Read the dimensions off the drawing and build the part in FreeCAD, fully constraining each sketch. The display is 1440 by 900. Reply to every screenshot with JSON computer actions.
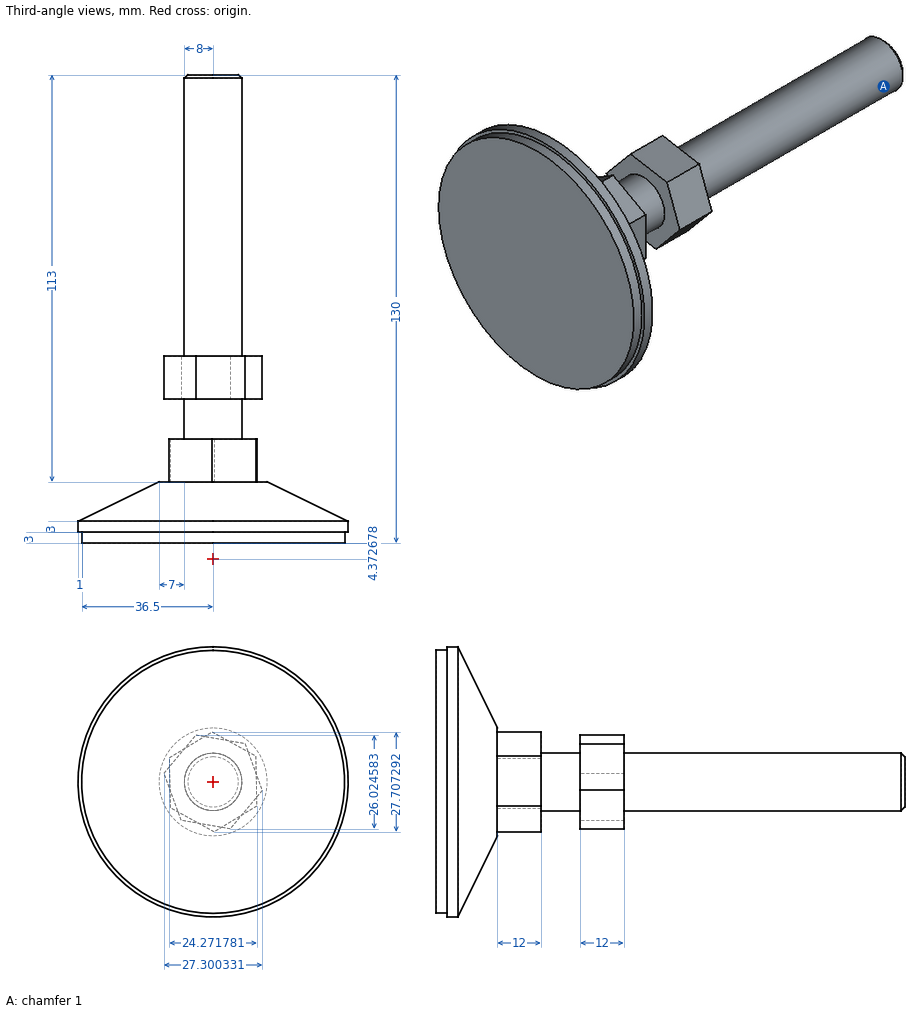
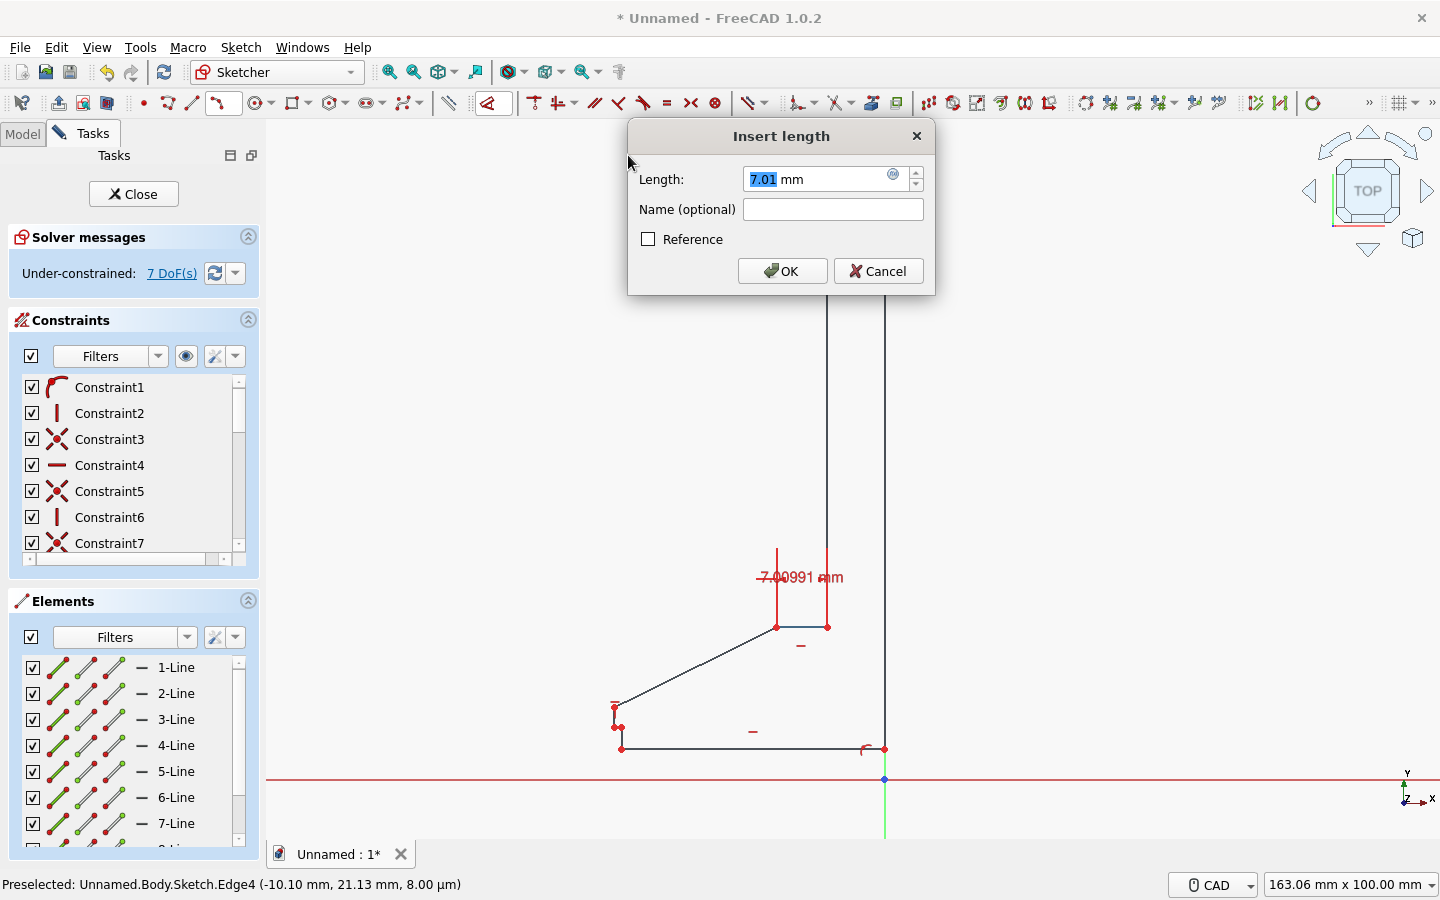
{"action": "type", "text": "7"}
{"action": "key", "text": "Return"}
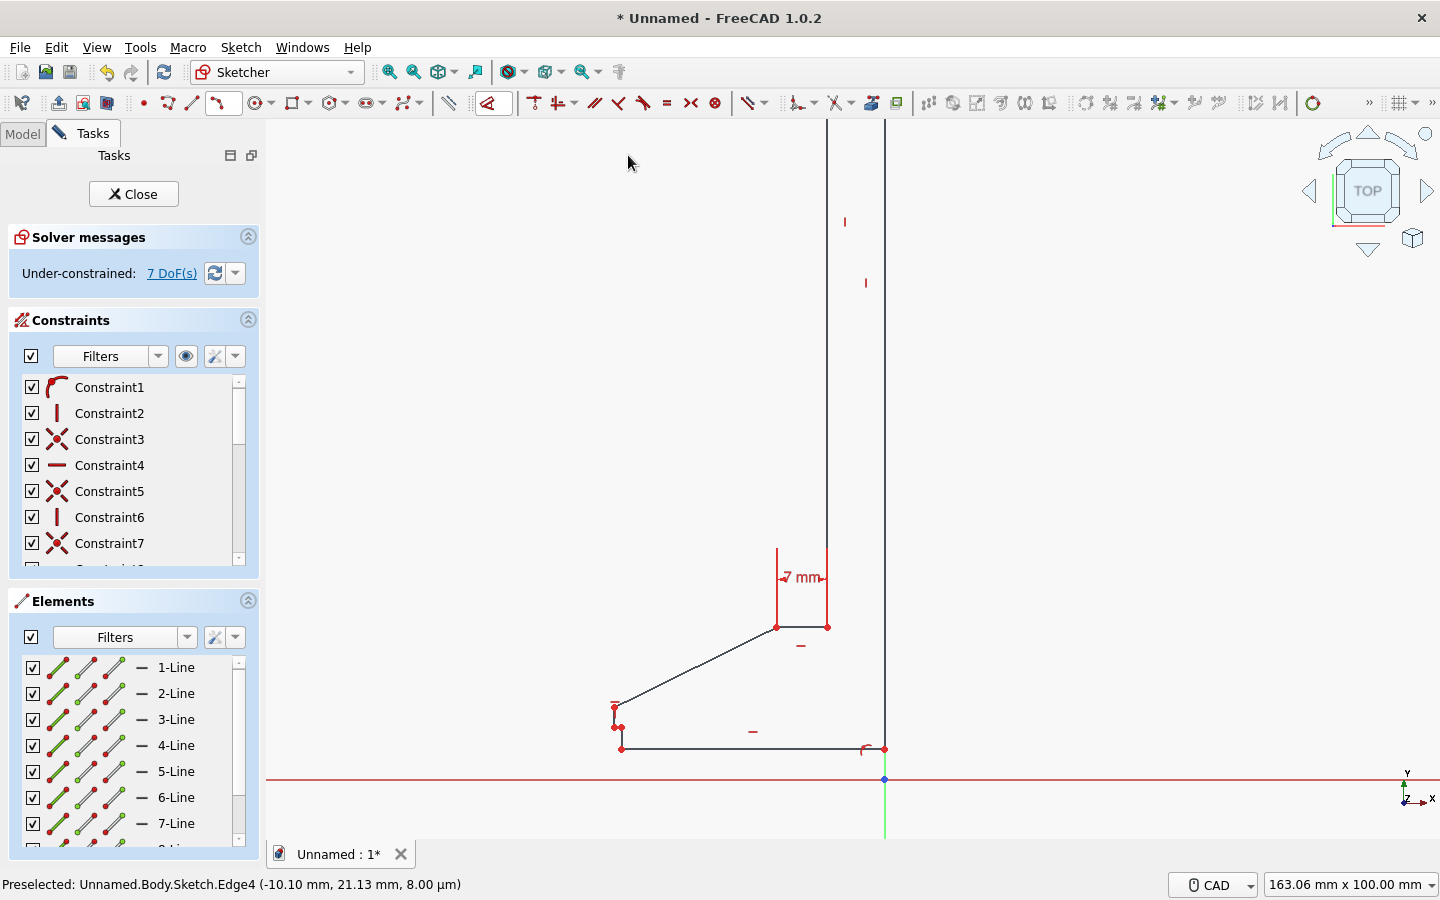
{"action": "scroll", "coordinate": [614, 717], "scroll_direction": "up", "scroll_amount": 4}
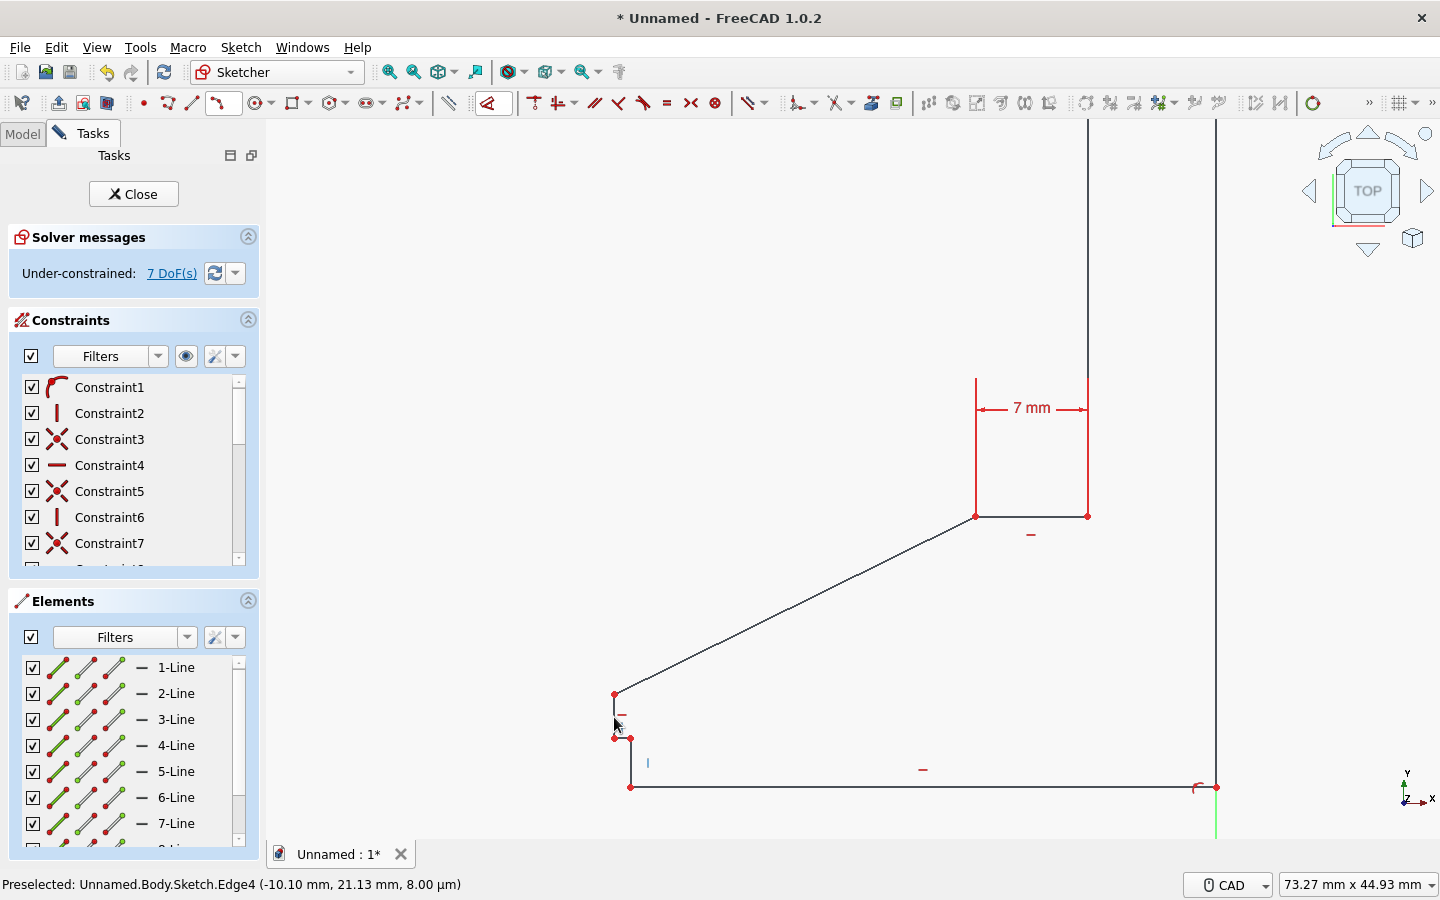
{"action": "left_click", "coordinate": [614, 717]}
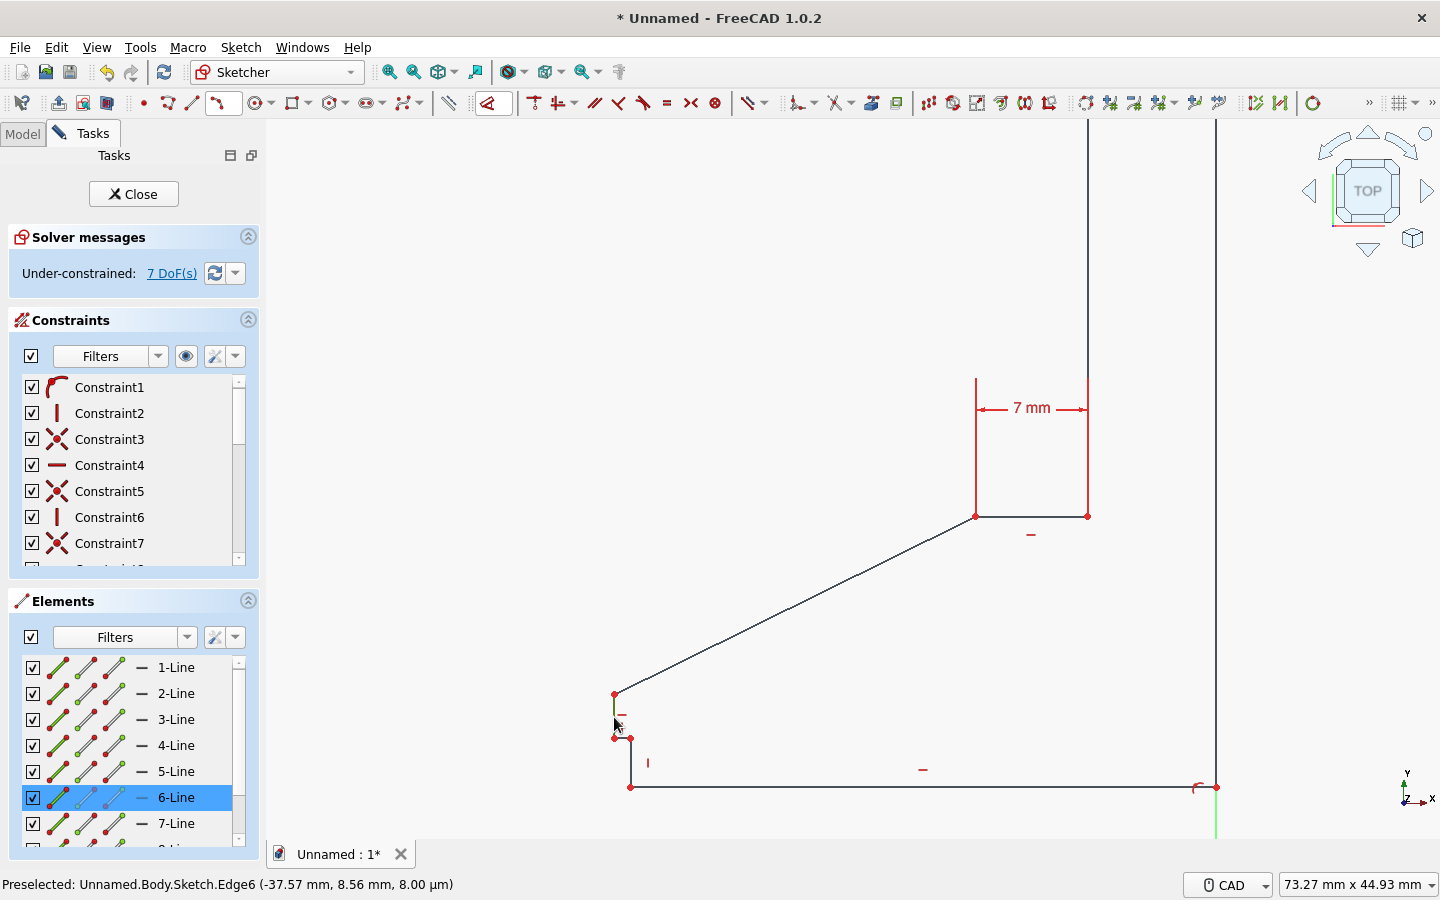
{"action": "key", "text": "i"}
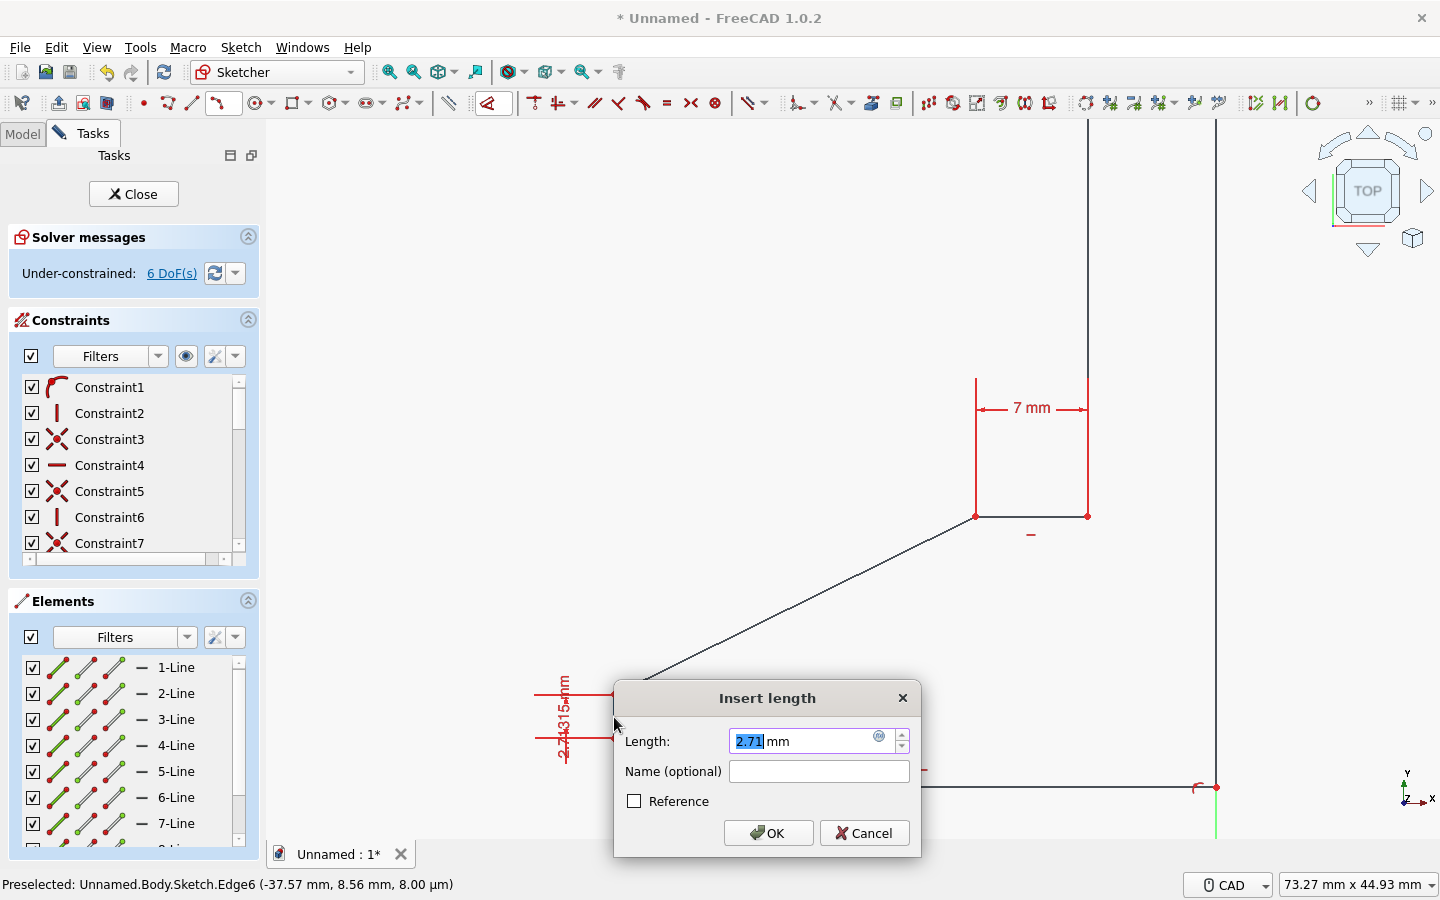
{"action": "type", "text": "3"}
{"action": "key", "text": "Return"}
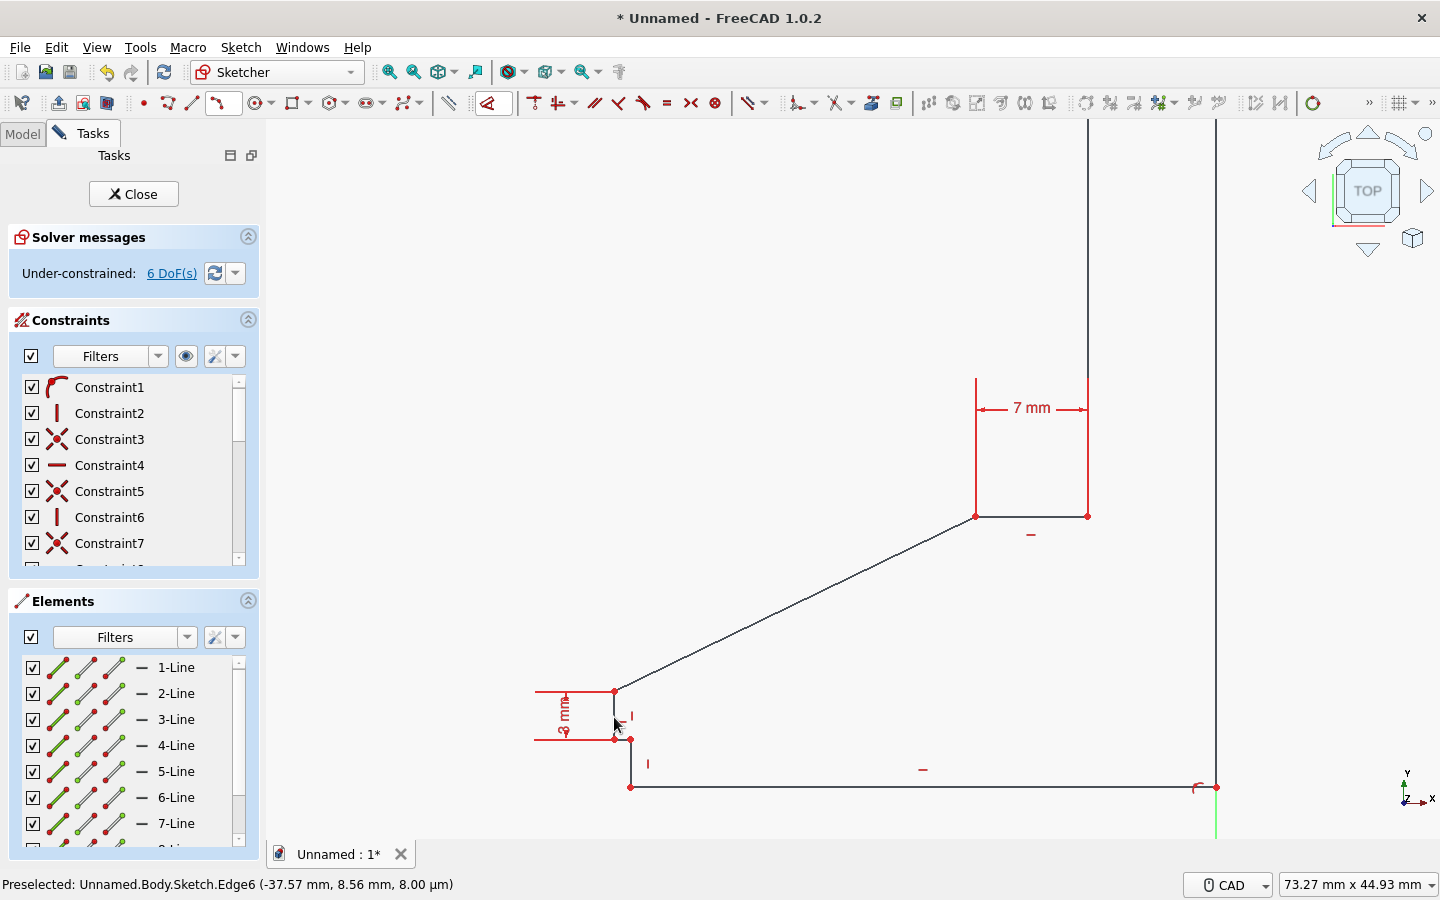
{"action": "scroll", "coordinate": [622, 740], "scroll_direction": "up", "scroll_amount": 5}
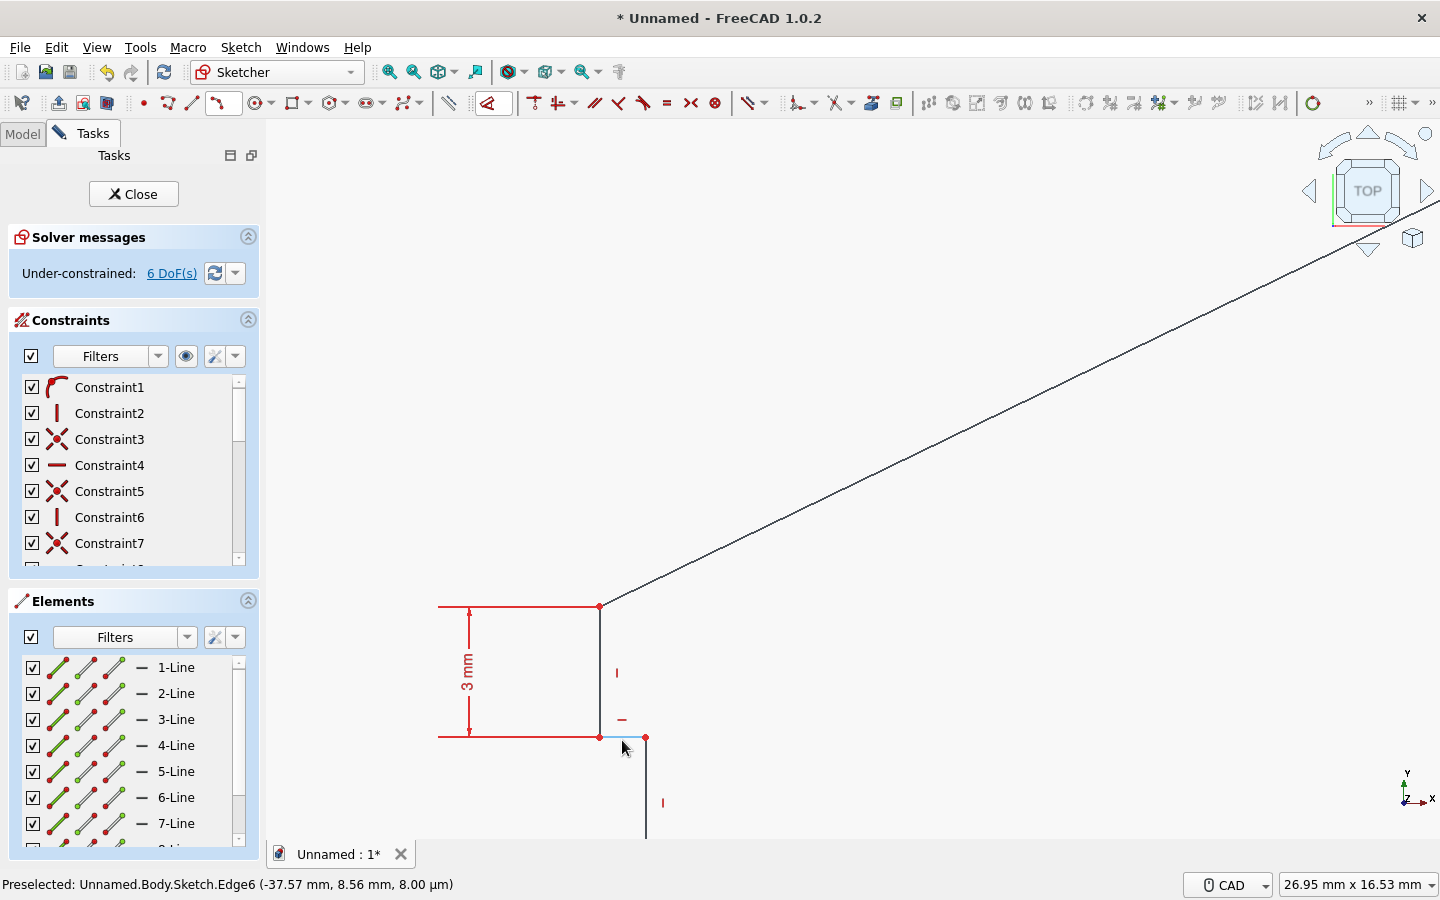
{"action": "left_click", "coordinate": [623, 737]}